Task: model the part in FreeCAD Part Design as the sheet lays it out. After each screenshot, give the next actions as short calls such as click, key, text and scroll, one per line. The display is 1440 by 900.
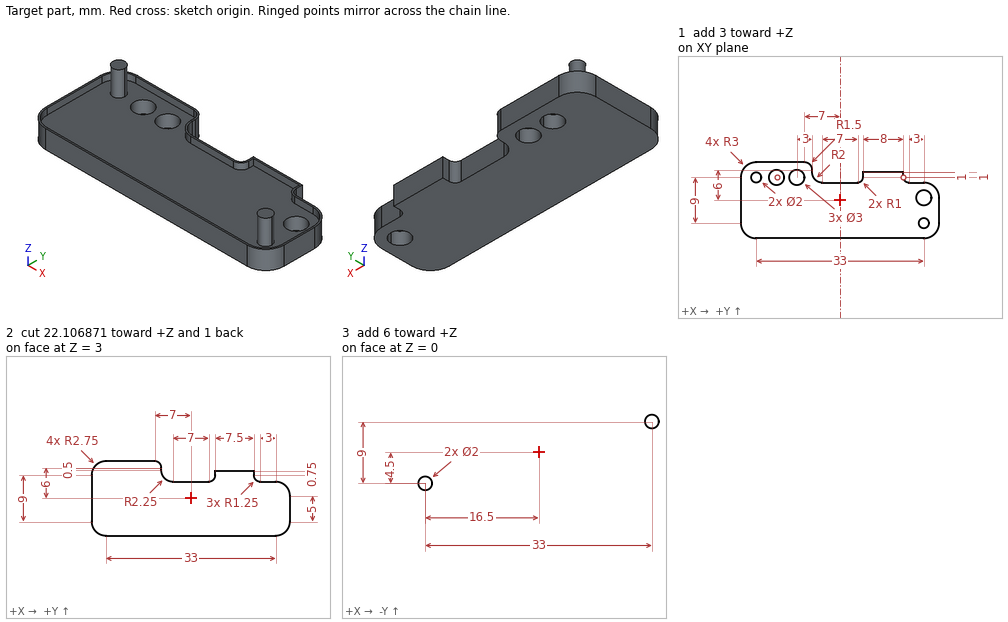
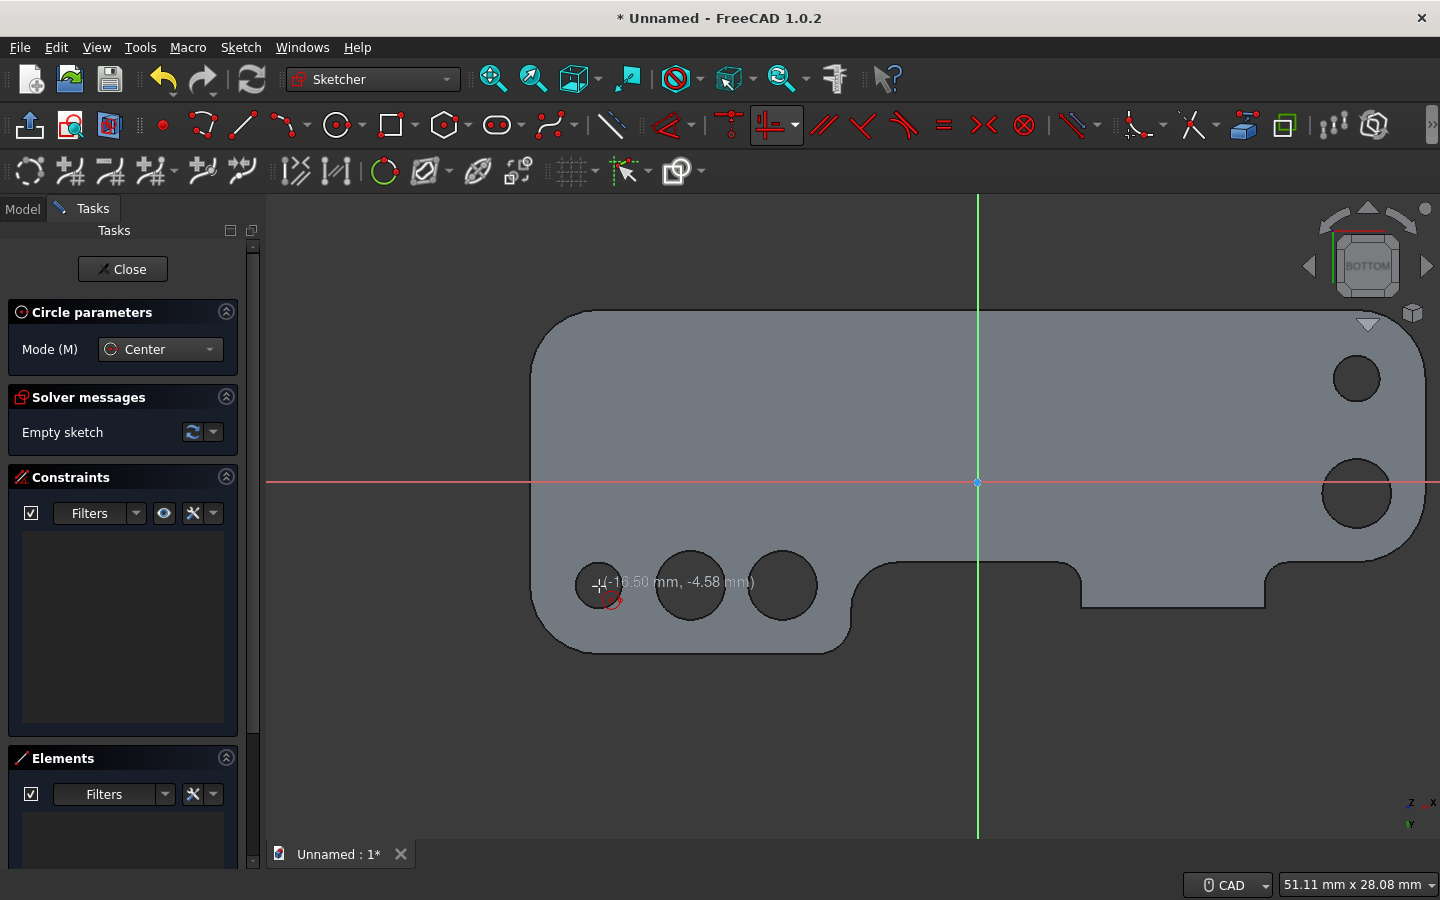
click(599, 585)
move(615, 569)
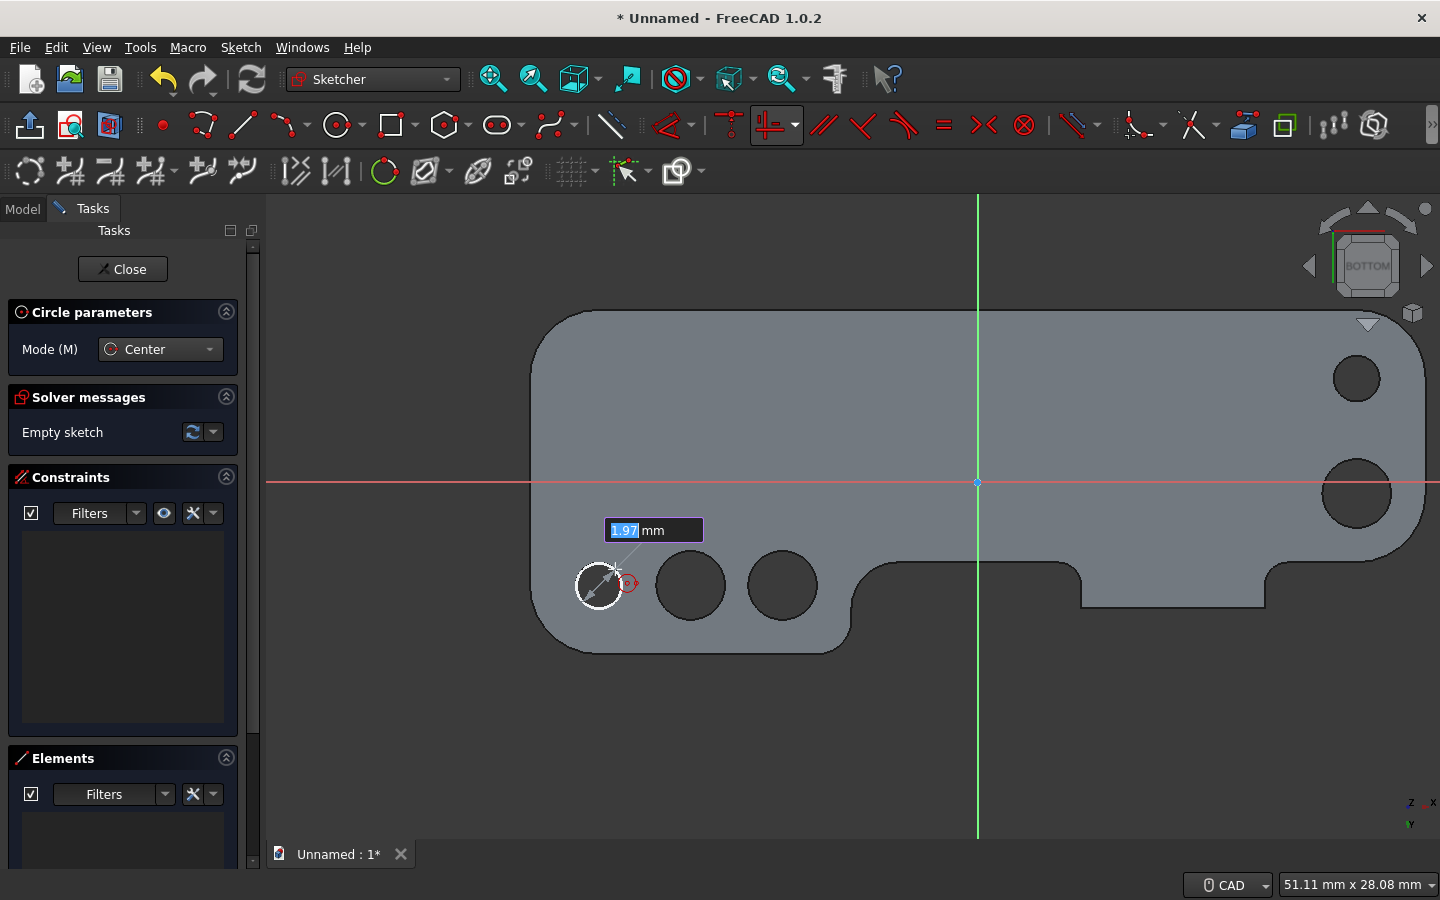
text(2)
key(Return)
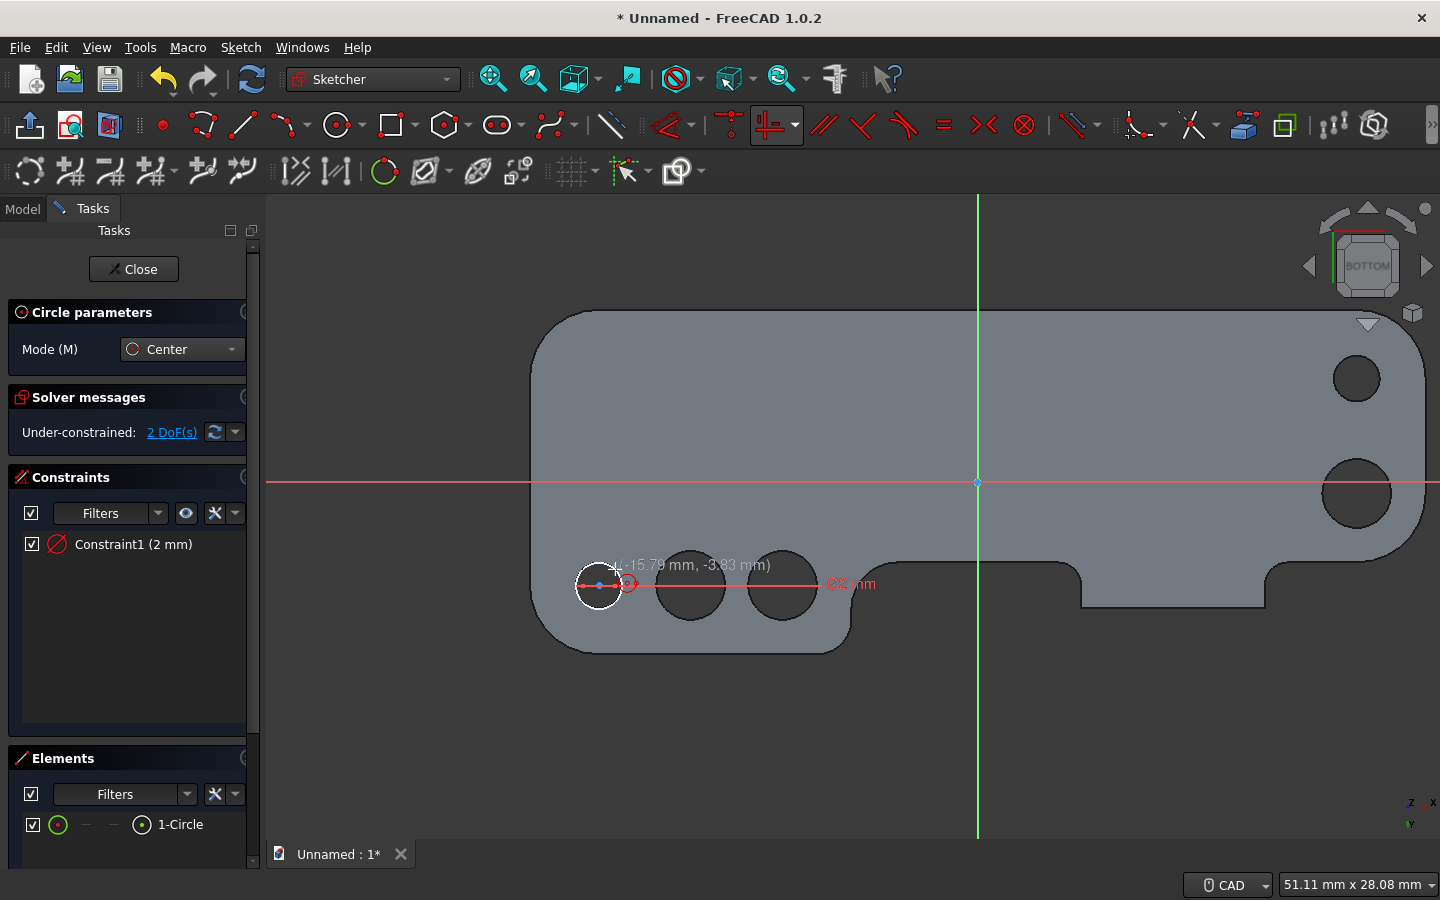
scroll(294, 672, down, 1)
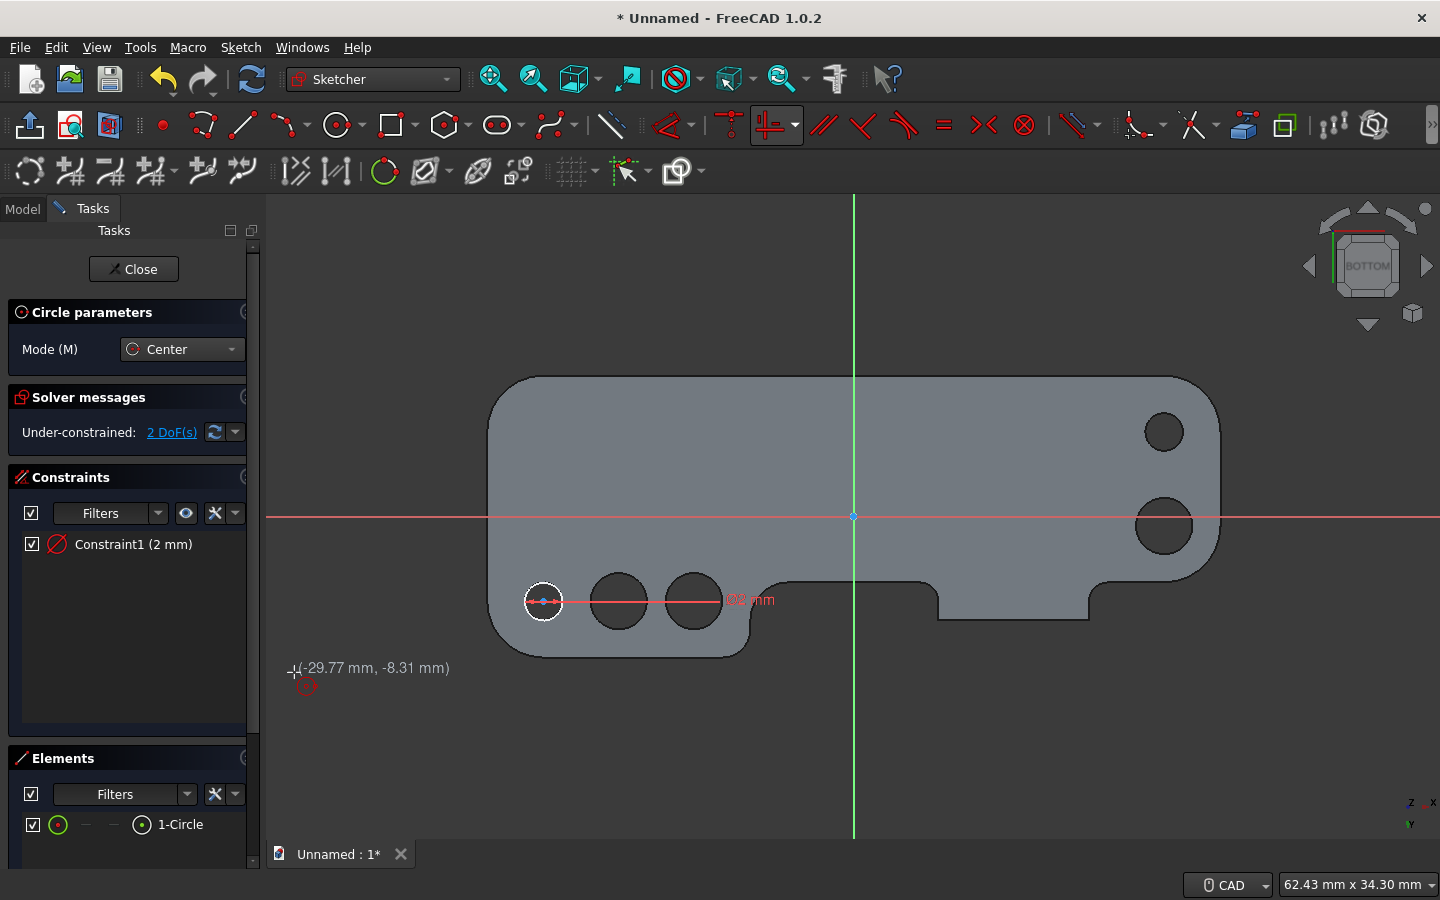
click(1164, 432)
move(1177, 419)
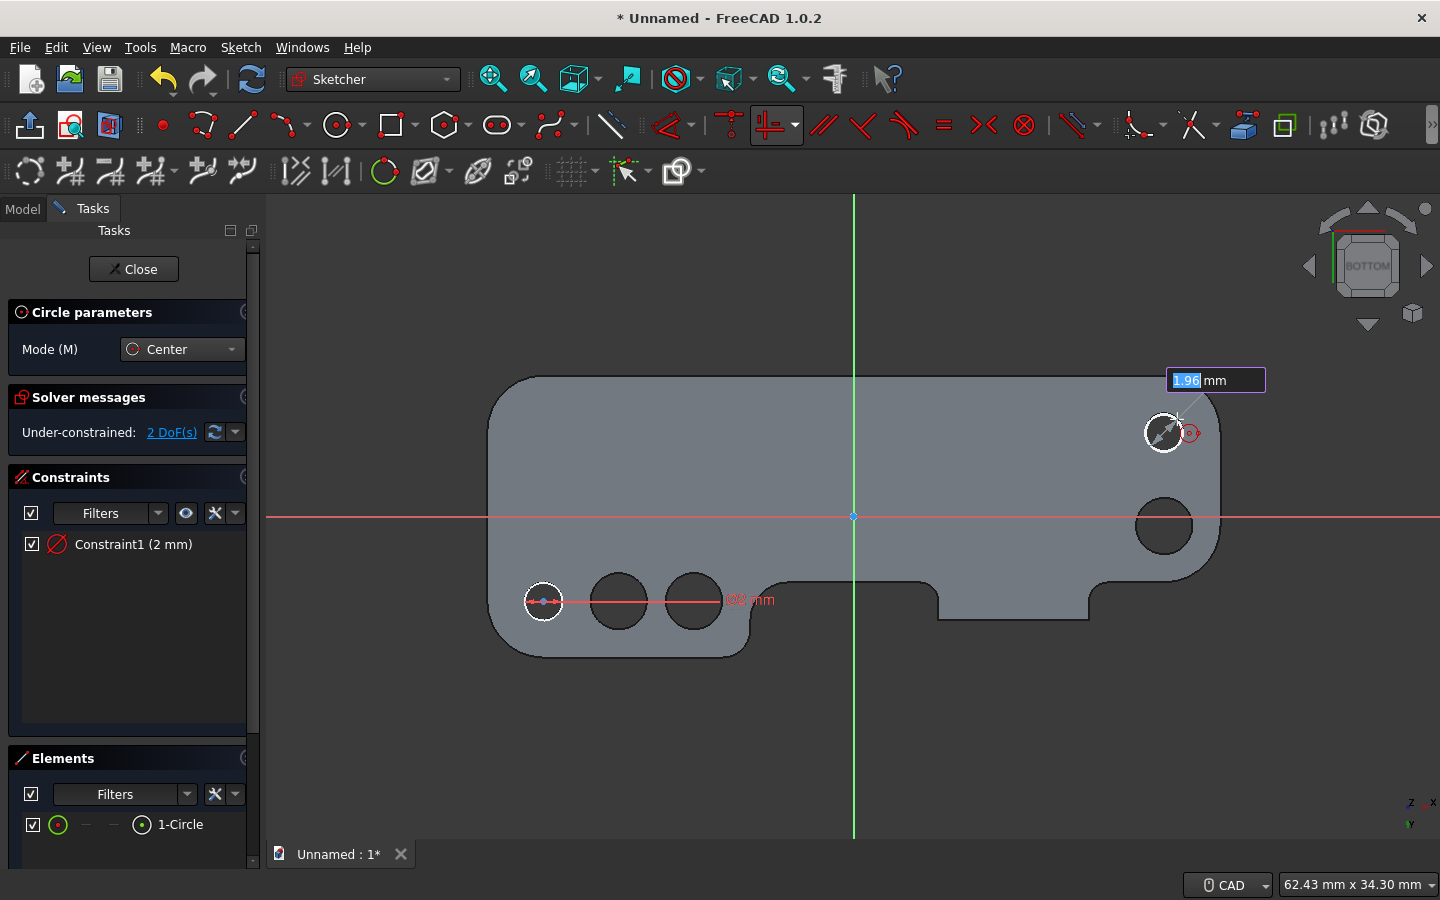
text(2)
key(Return)
key(Escape)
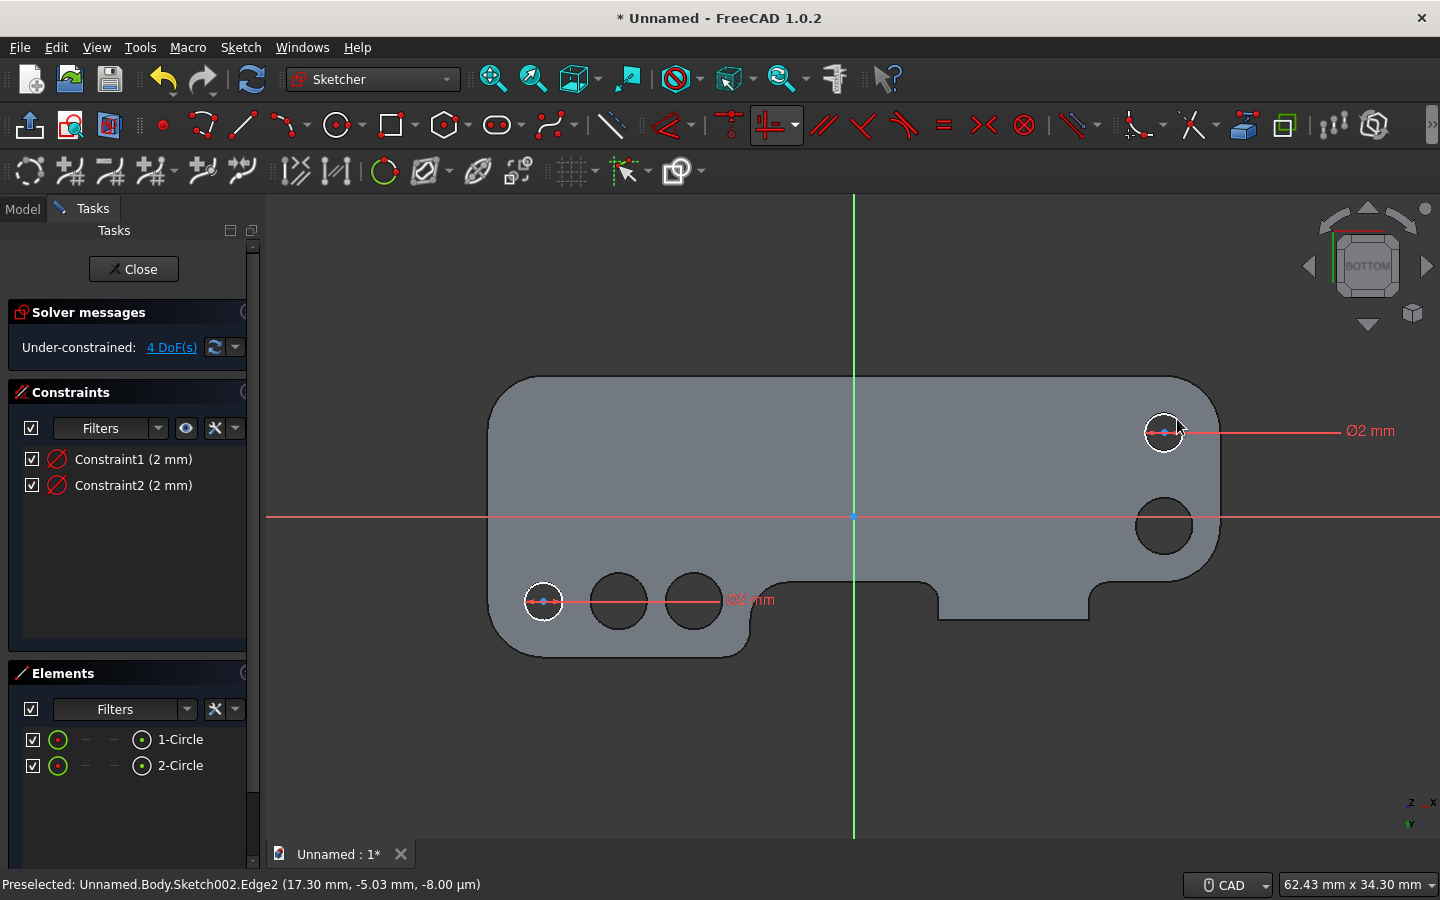
click(666, 126)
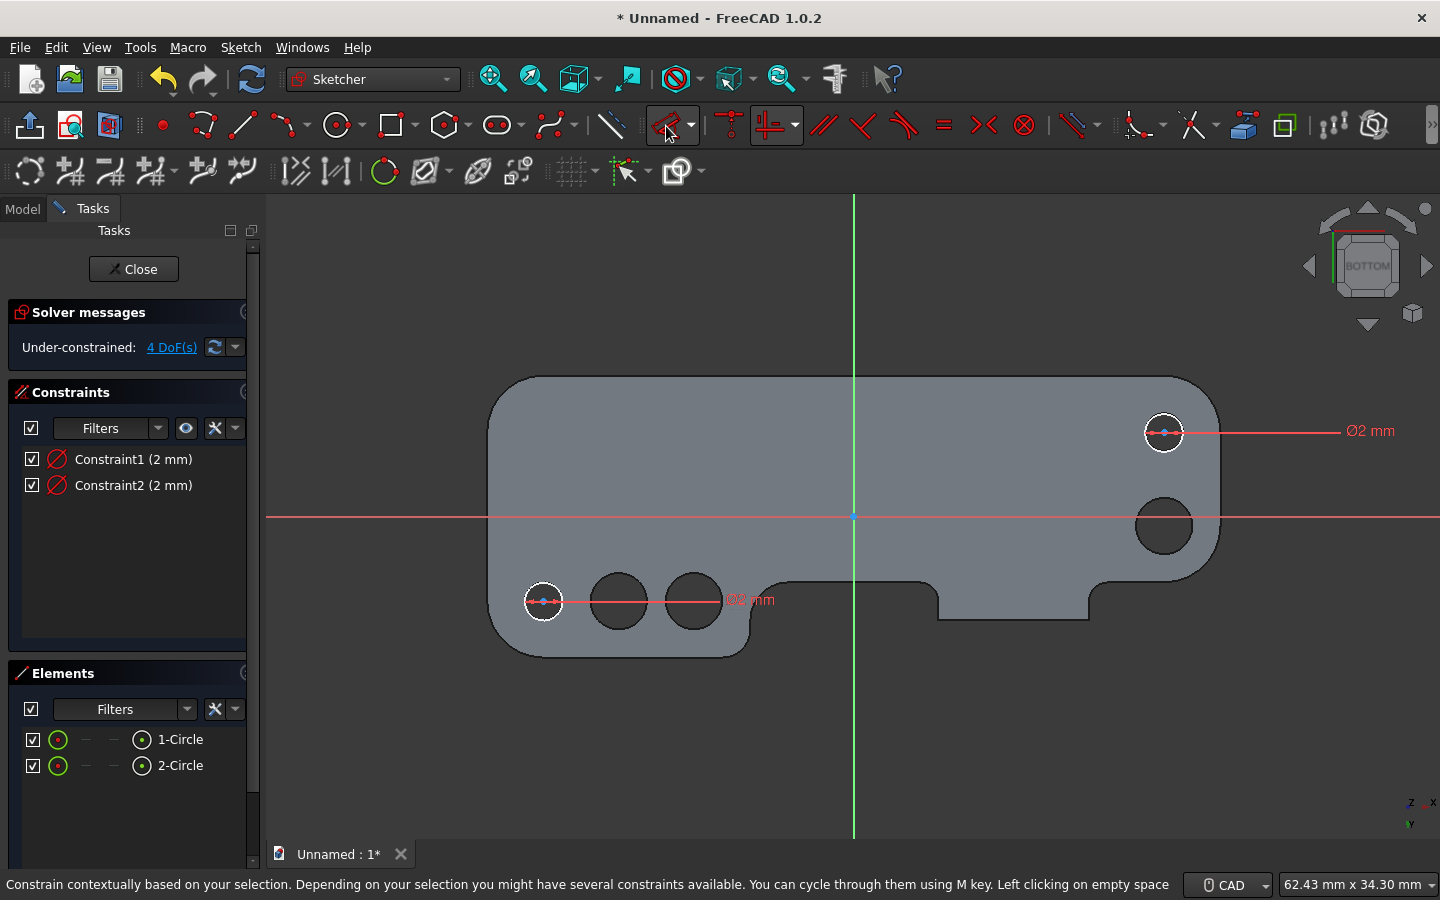
click(544, 602)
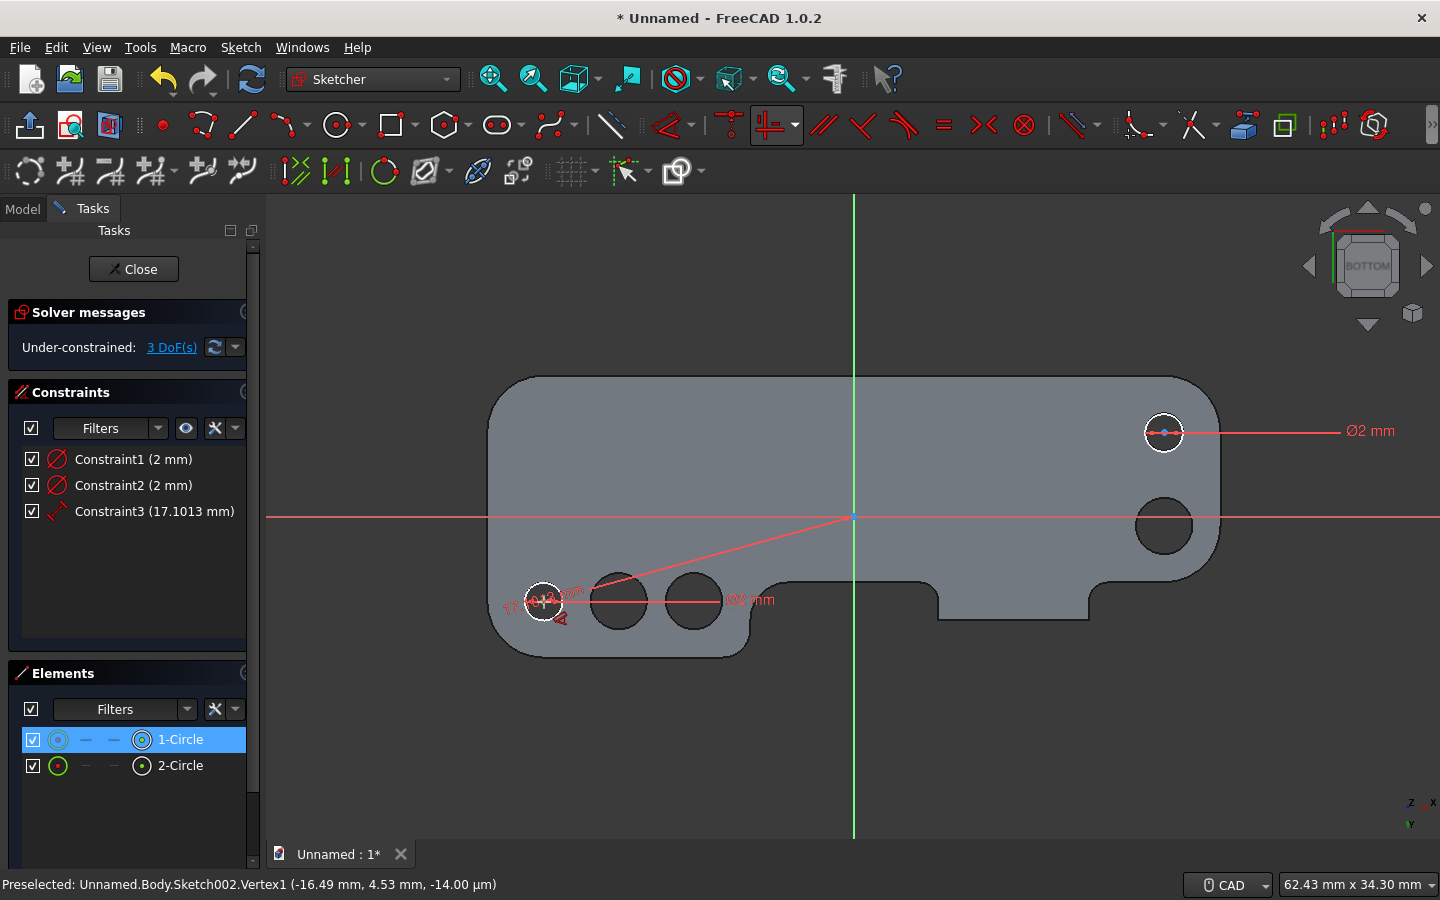
click(1164, 433)
click(1198, 479)